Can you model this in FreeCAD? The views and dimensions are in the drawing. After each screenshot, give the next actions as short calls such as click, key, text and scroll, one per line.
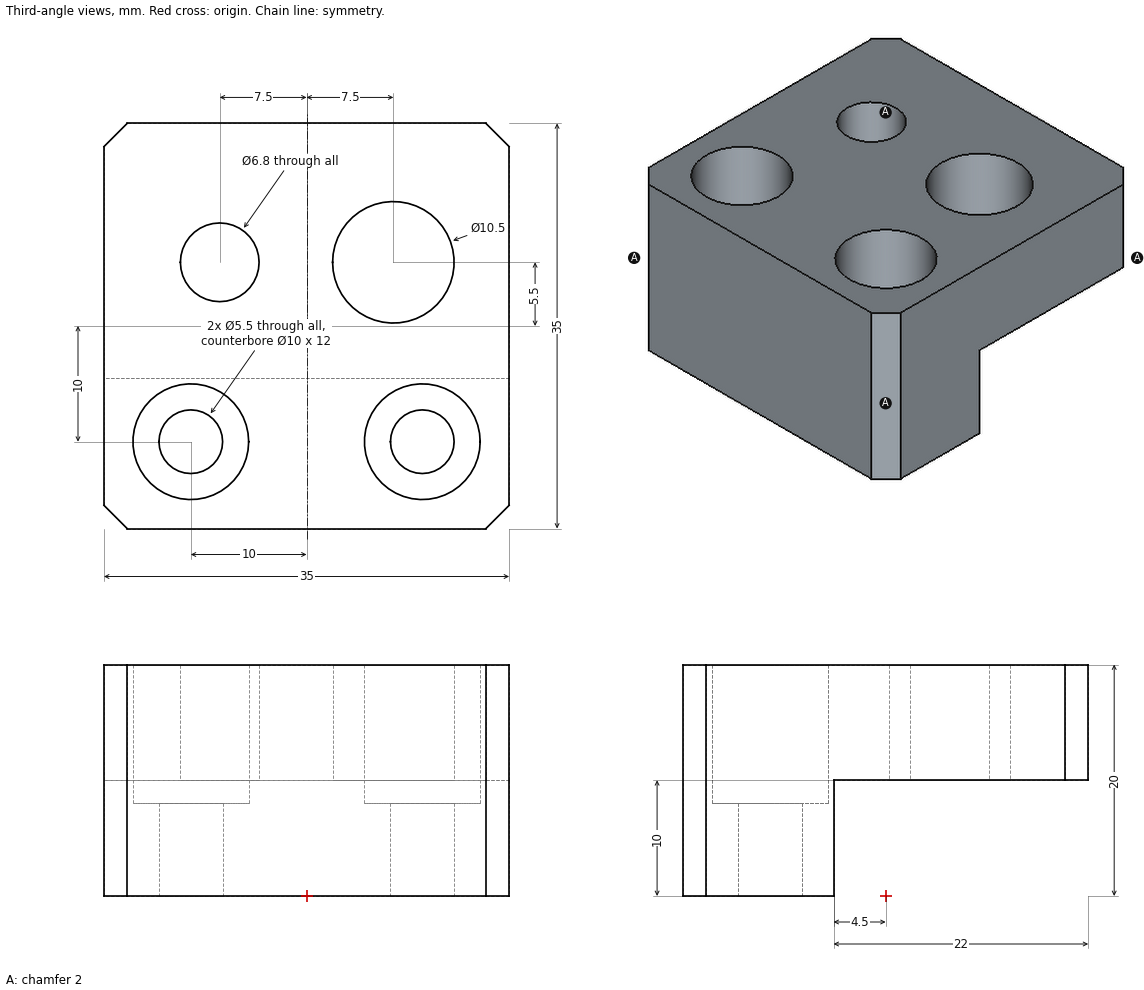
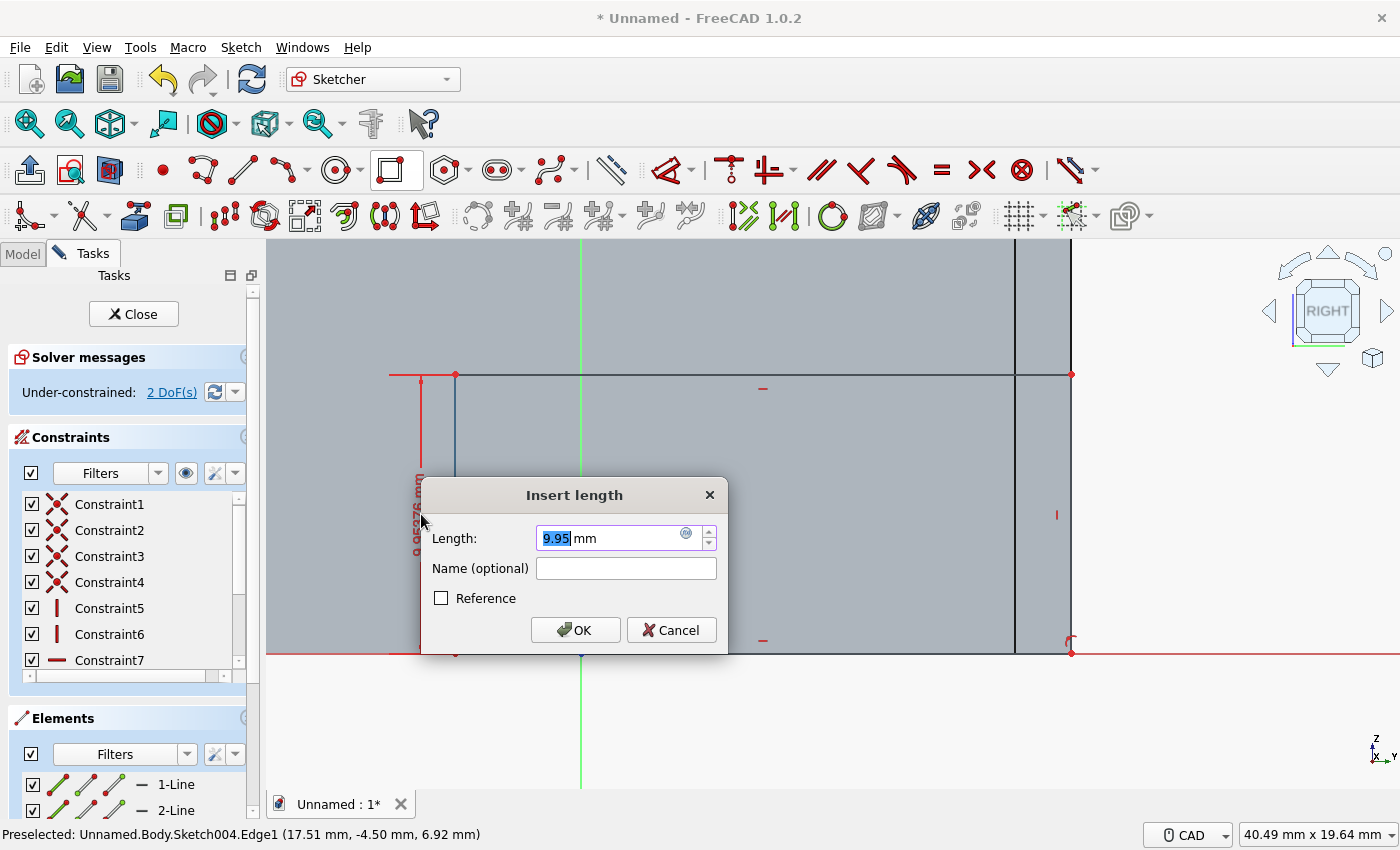
text(10)
key(Return)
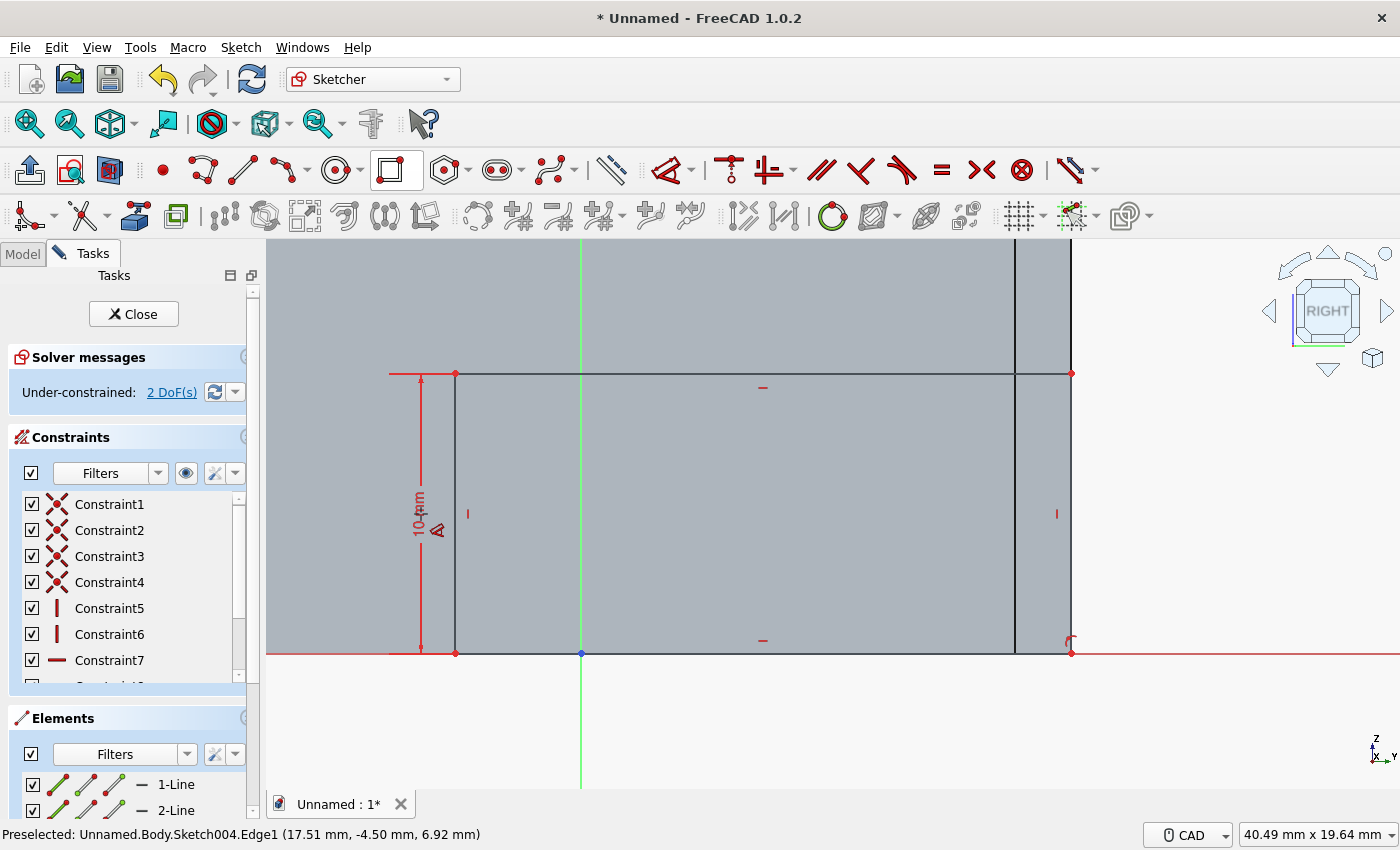
click(640, 654)
click(763, 688)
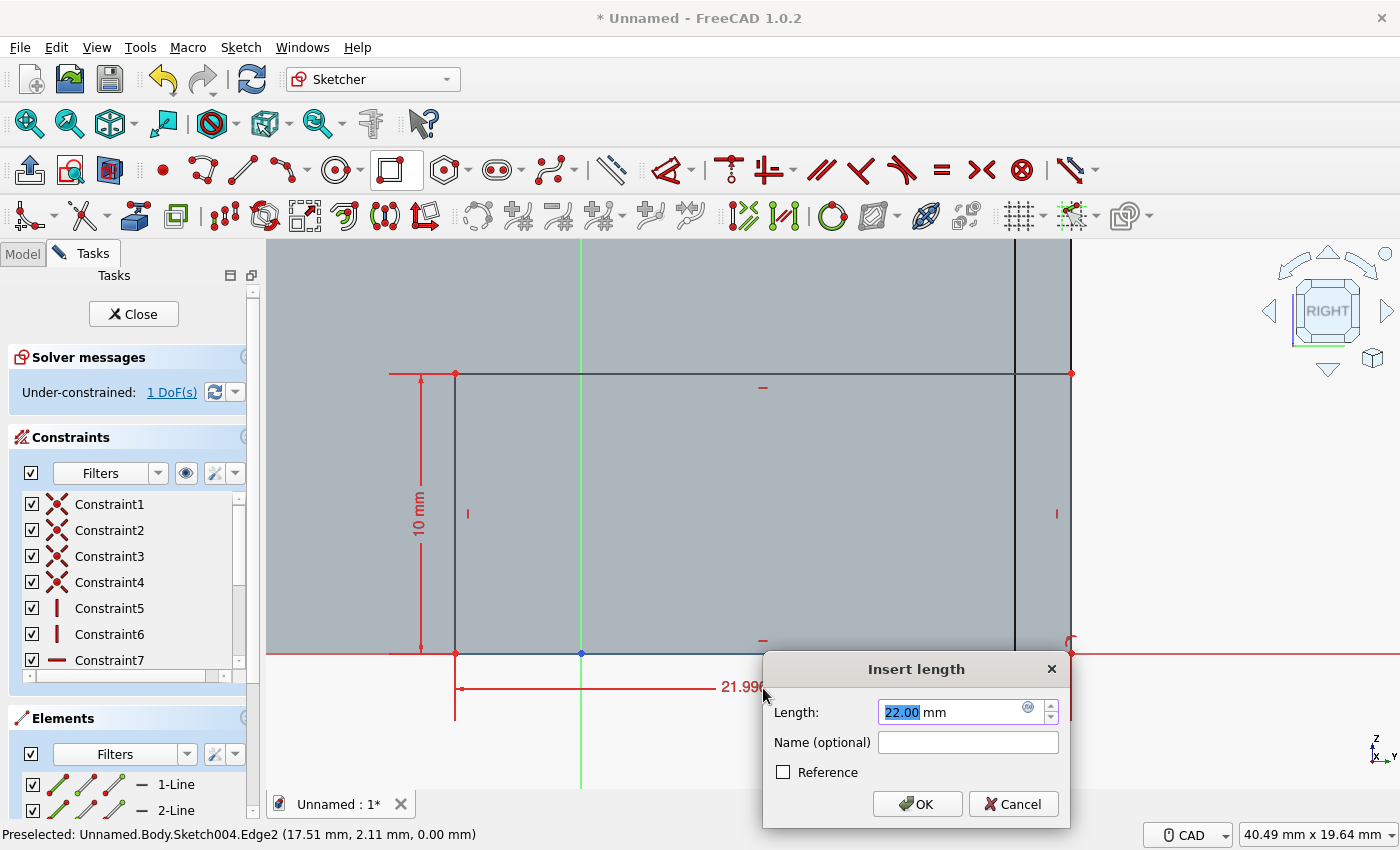
text(22)
key(Return)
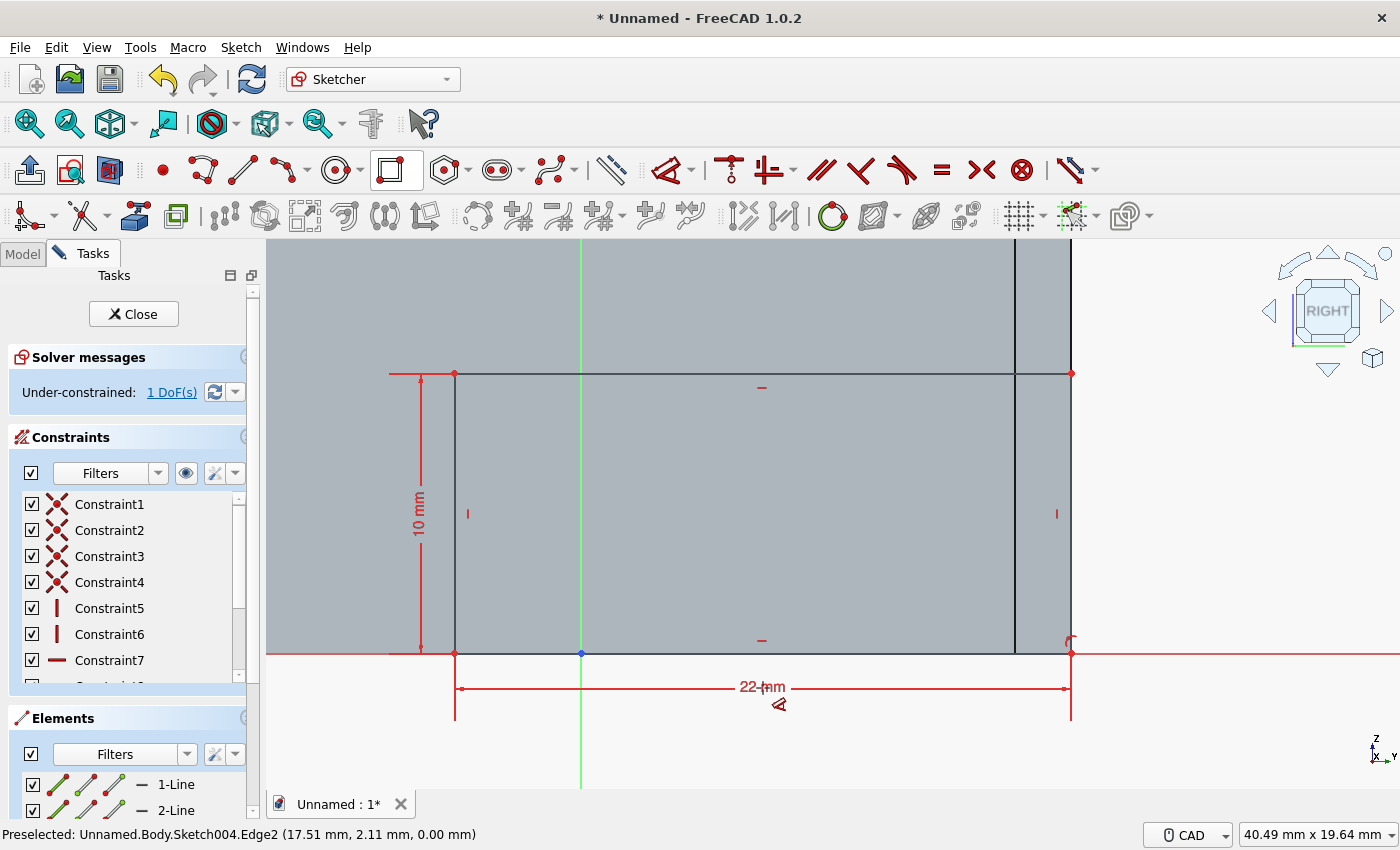
click(455, 374)
click(518, 688)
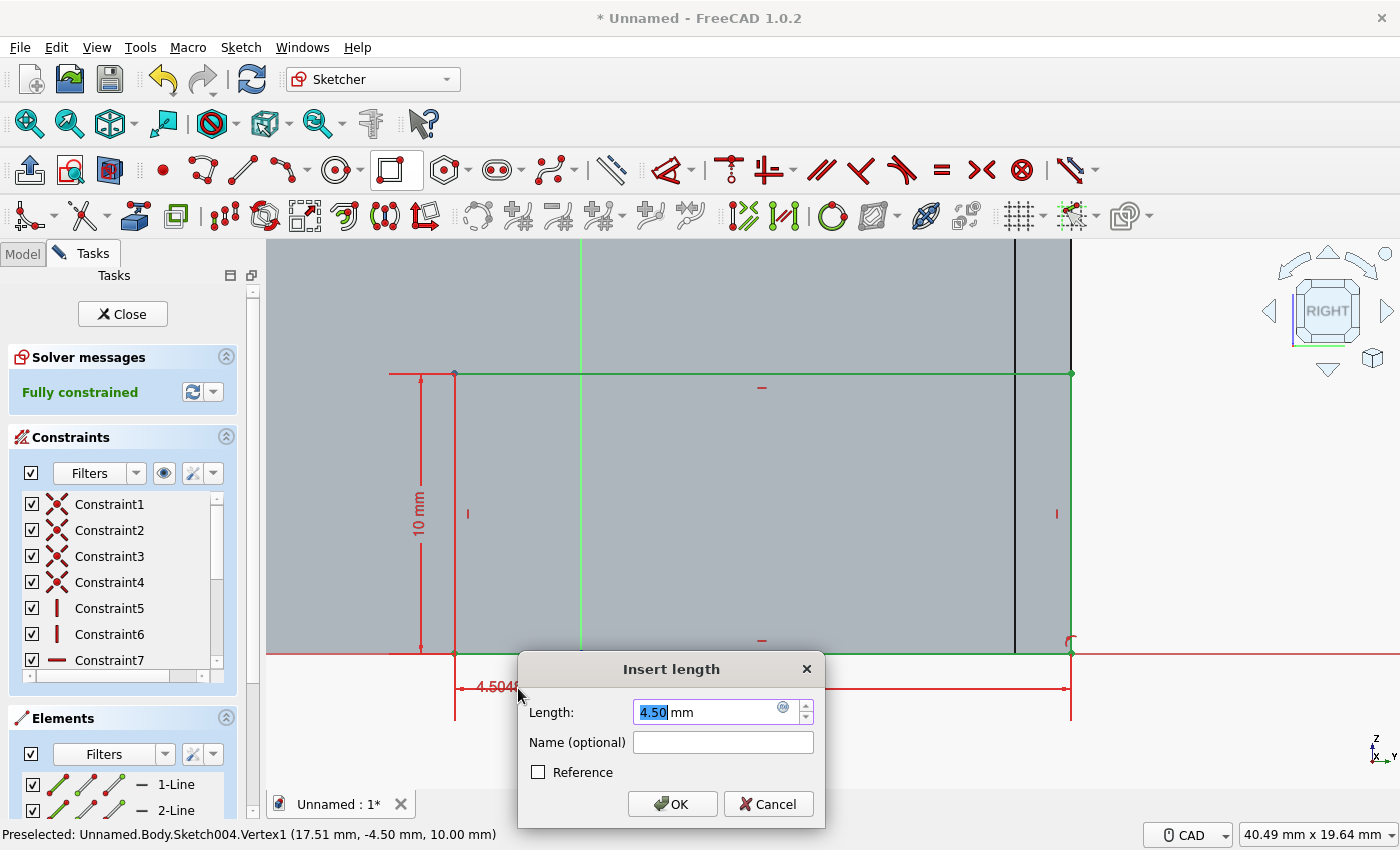
text(4.5)
key(Return)
key(Escape)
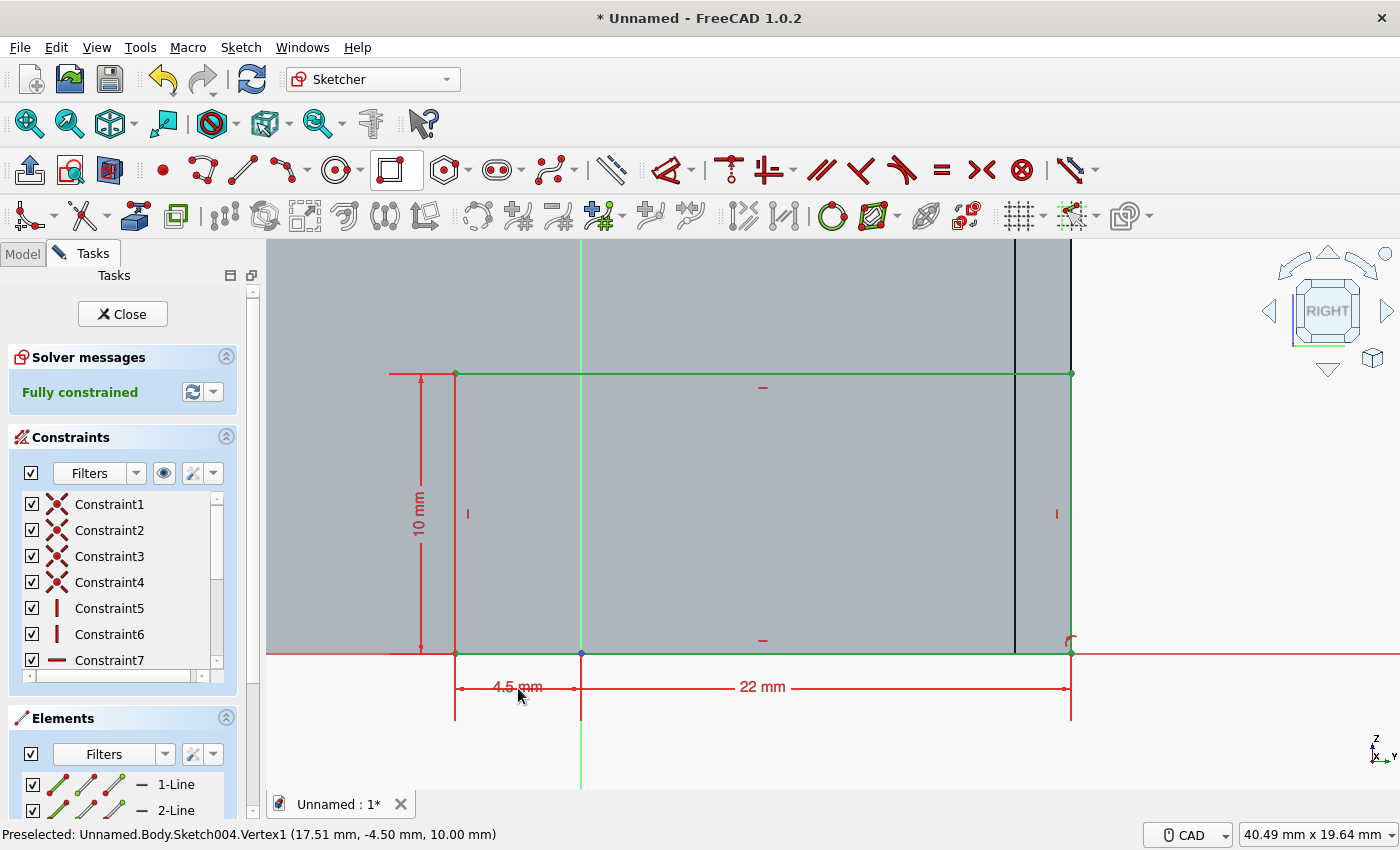
click(123, 314)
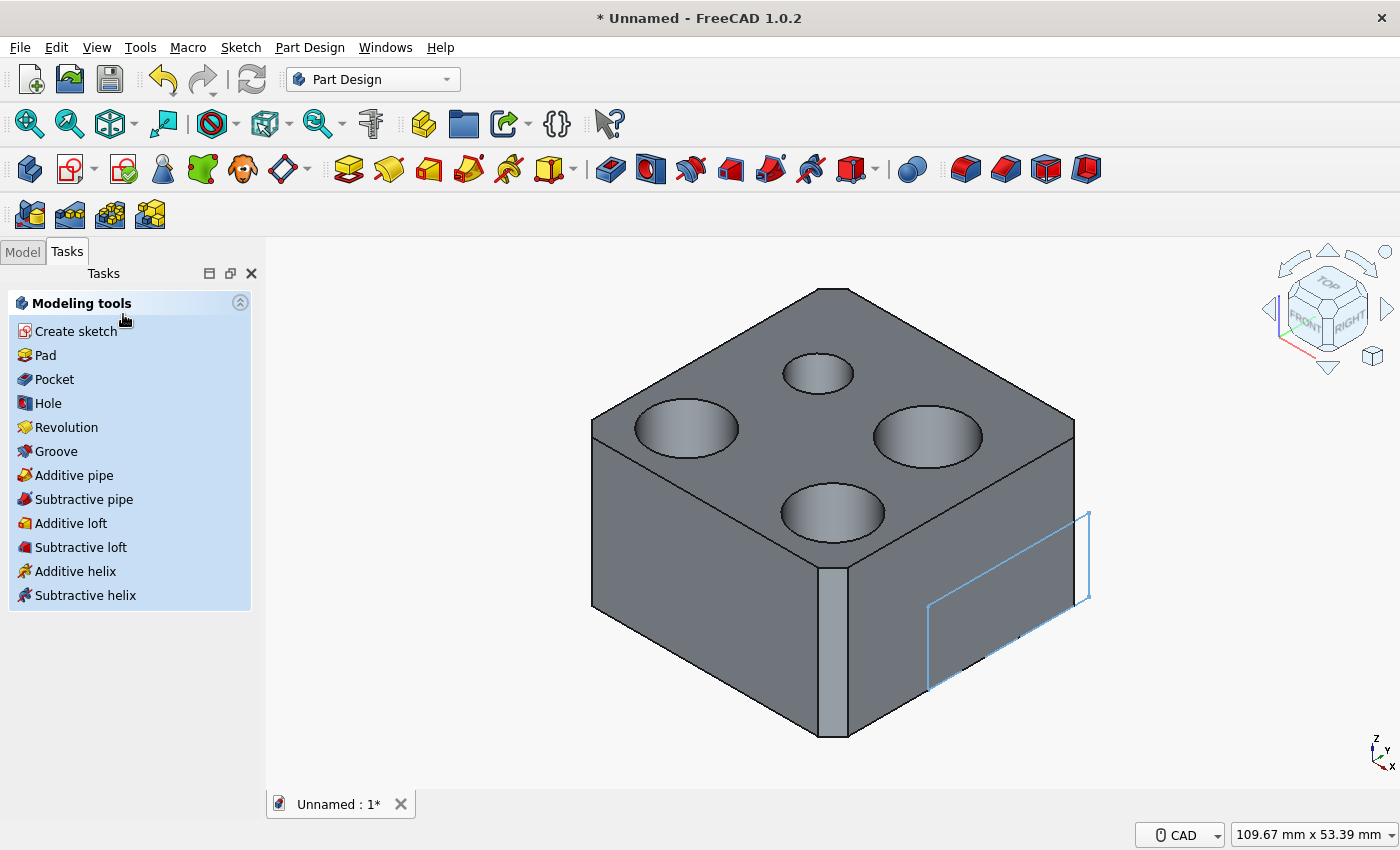
click(612, 170)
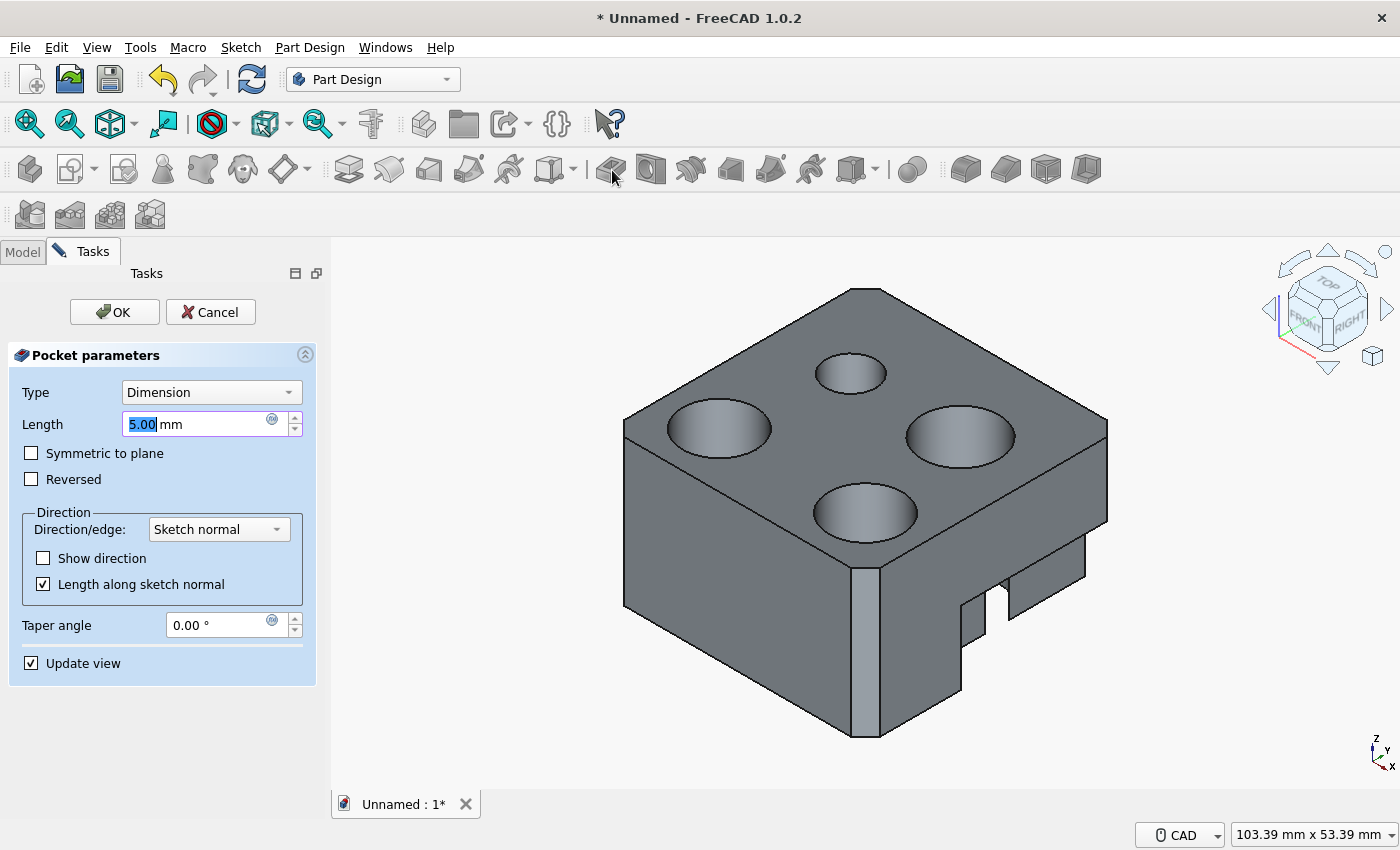
click(212, 392)